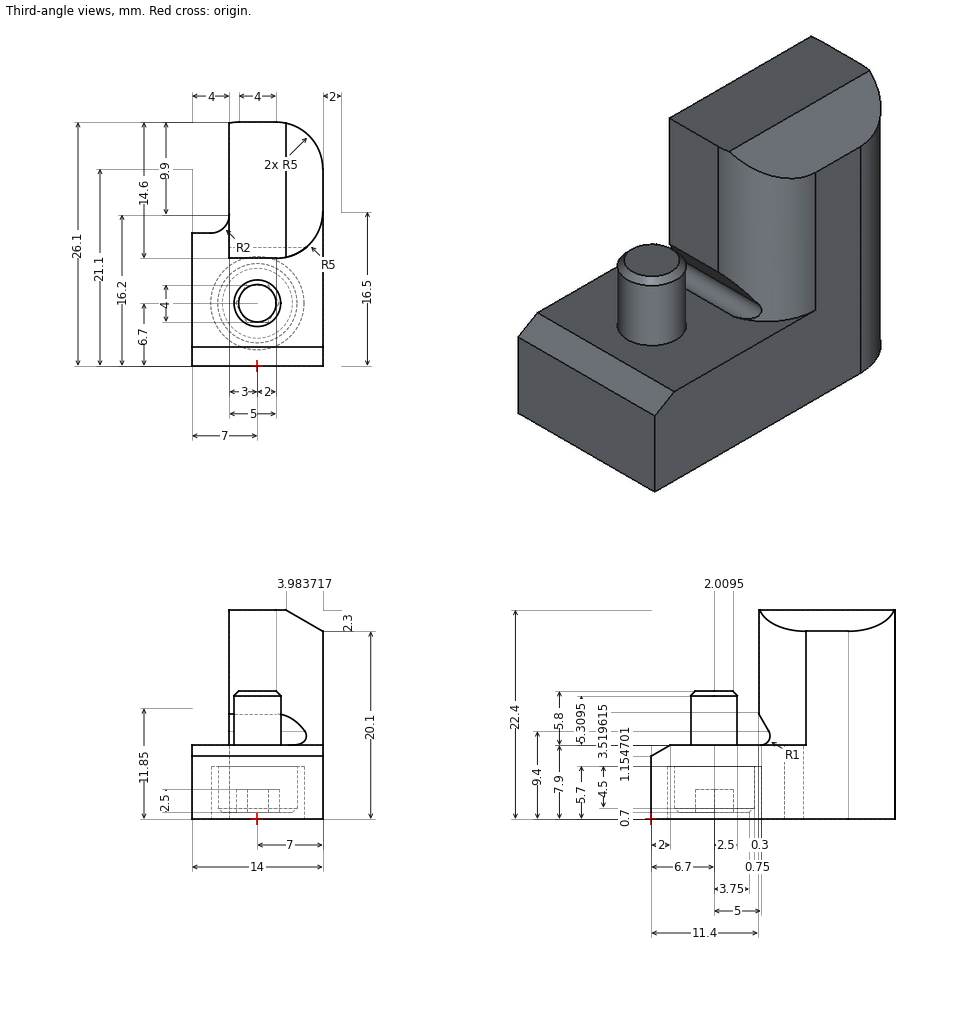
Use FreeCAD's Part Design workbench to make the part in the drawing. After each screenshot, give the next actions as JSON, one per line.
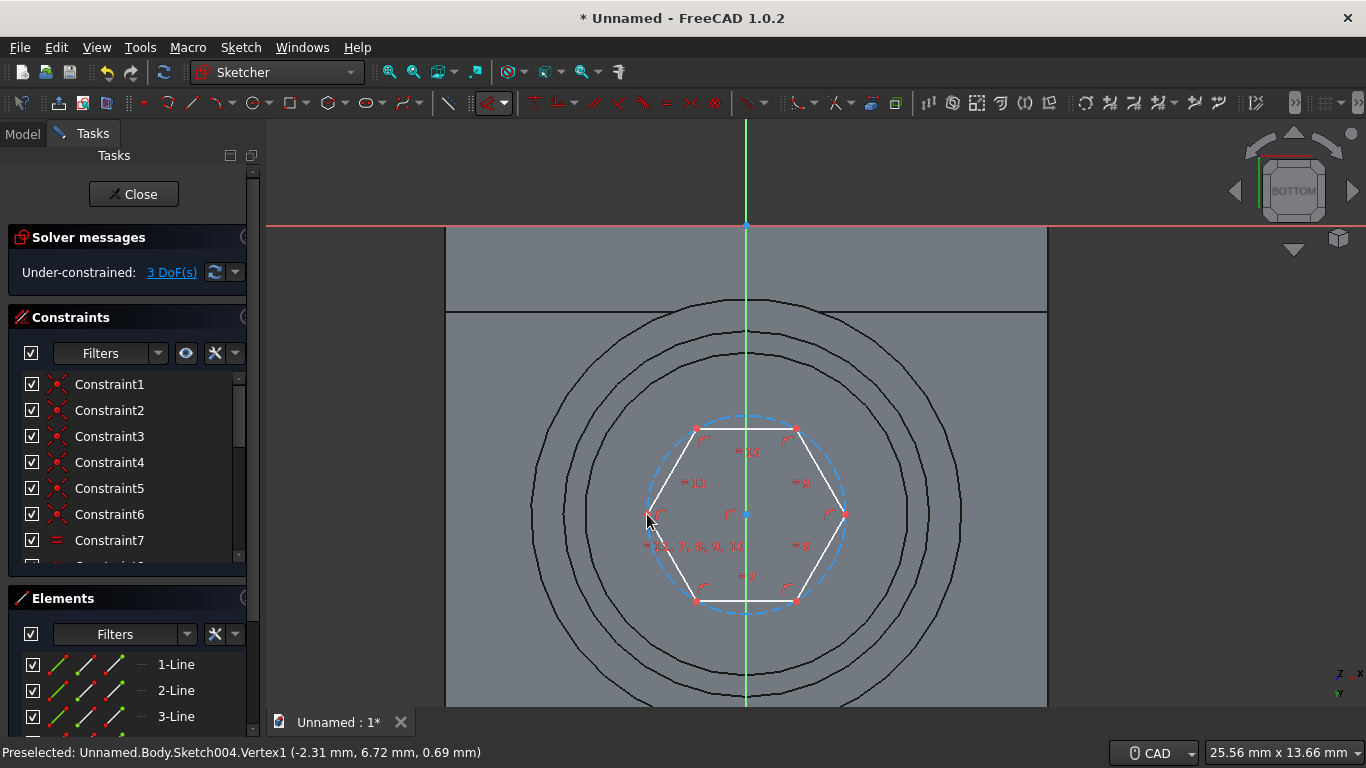
{"action": "scroll", "coordinate": [726, 601], "scroll_direction": "up", "scroll_amount": 2}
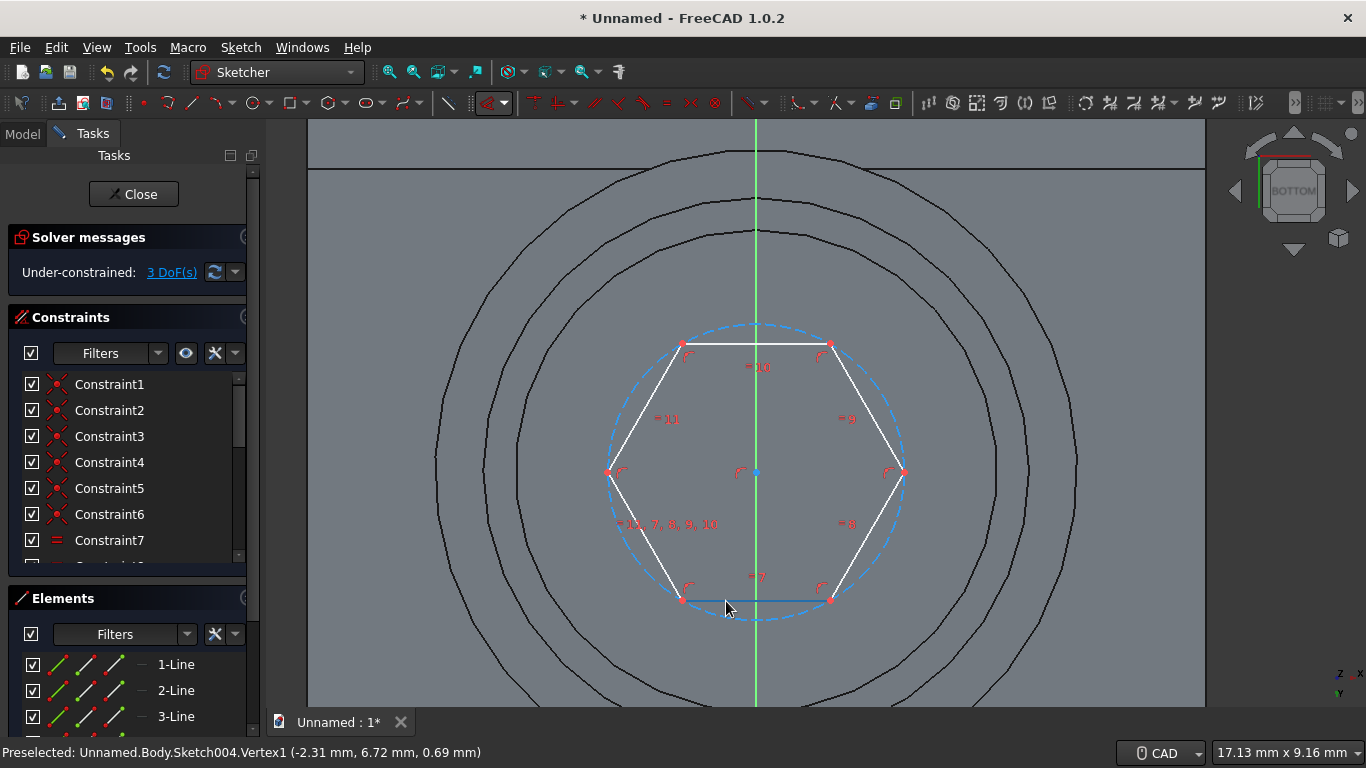
{"action": "left_click", "coordinate": [727, 601]}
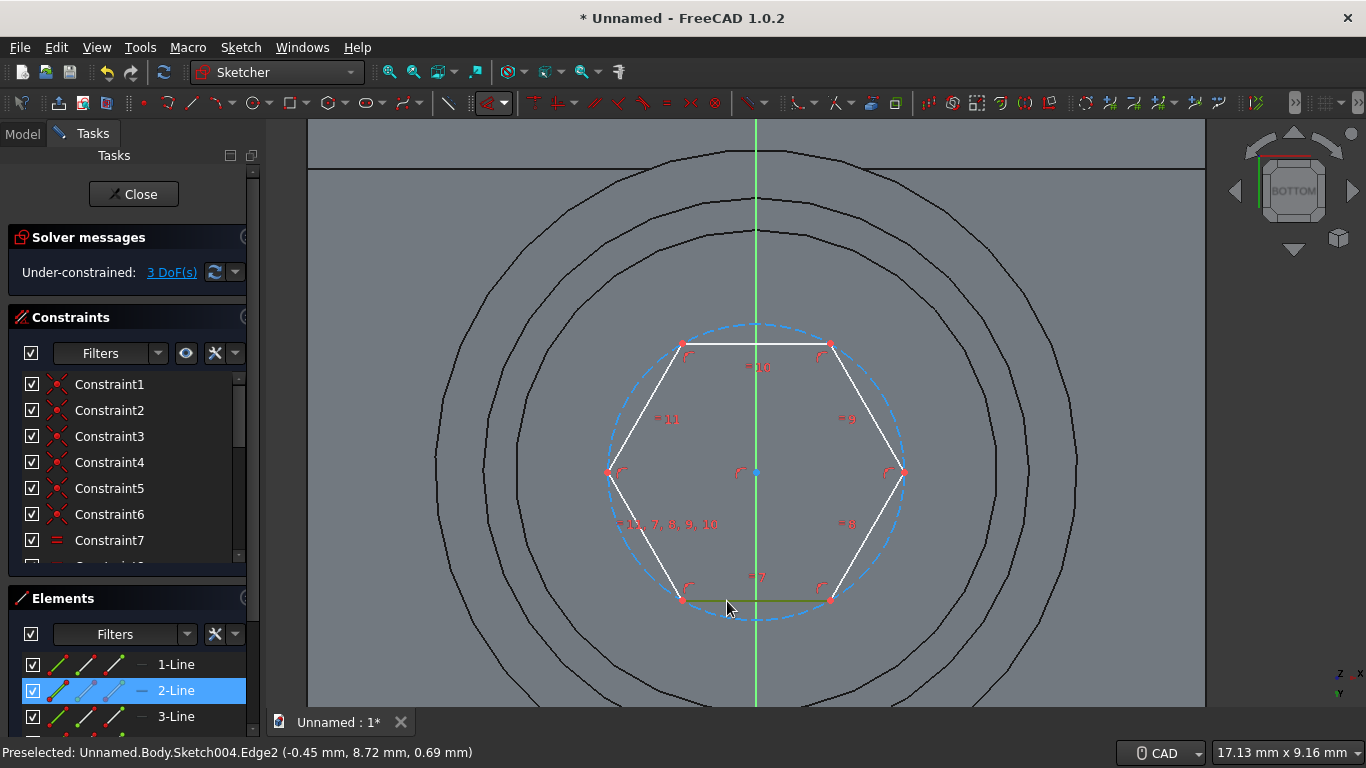
{"action": "key", "text": "h"}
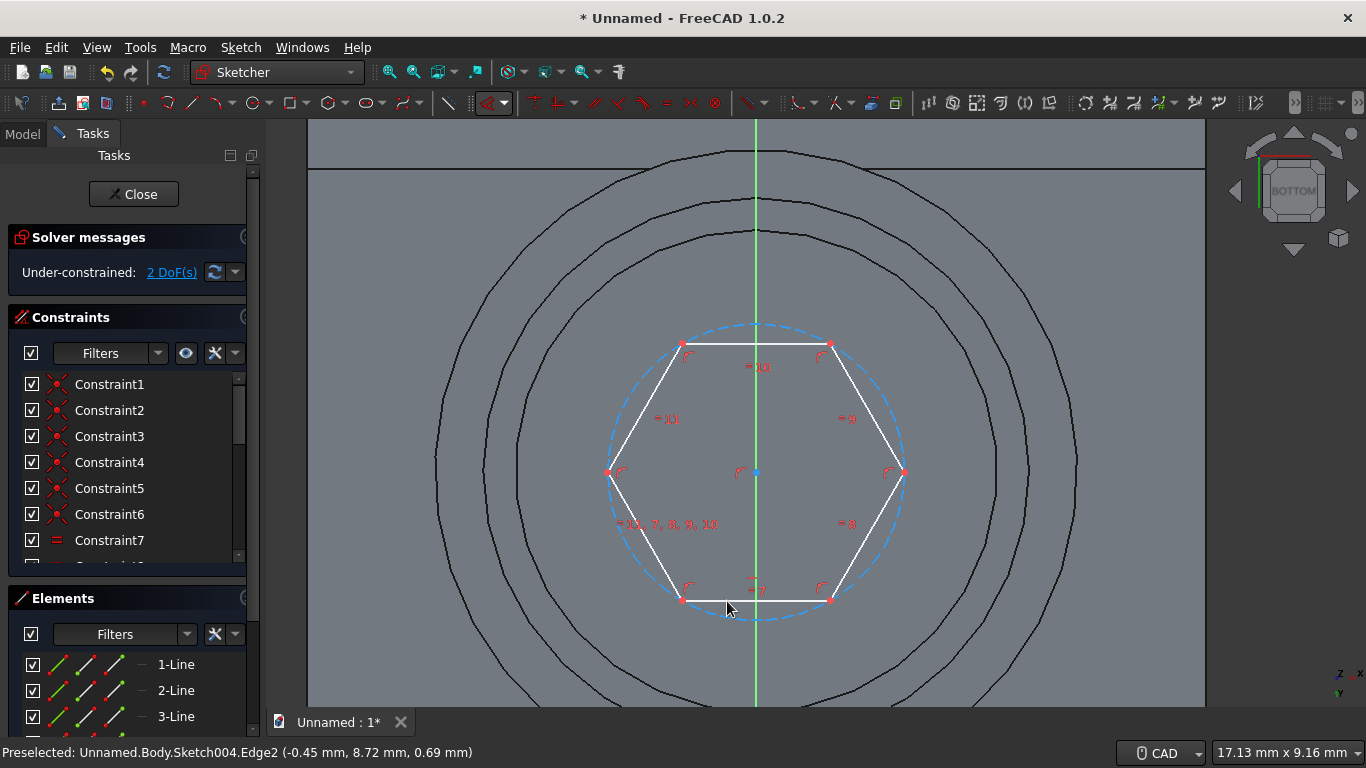
{"action": "left_click", "coordinate": [682, 601]}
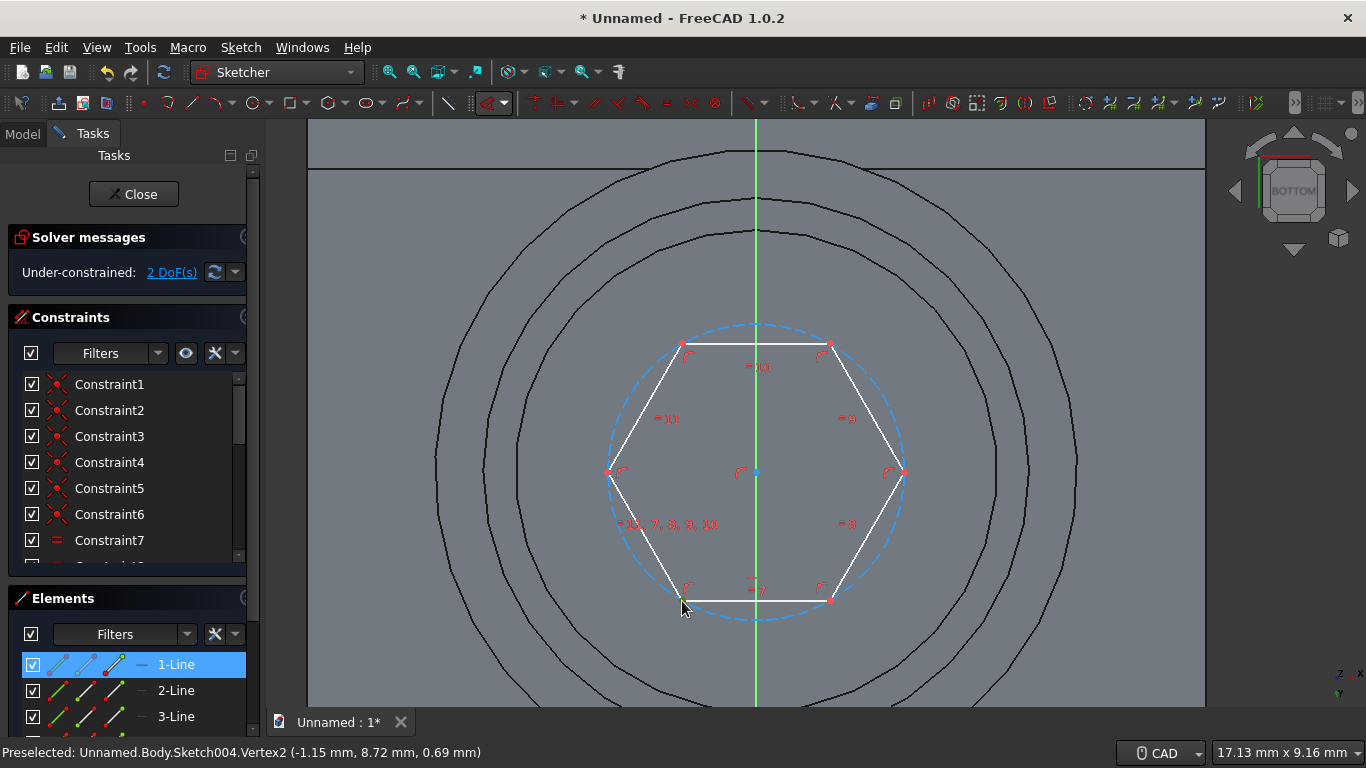
{"action": "left_click", "coordinate": [830, 344]}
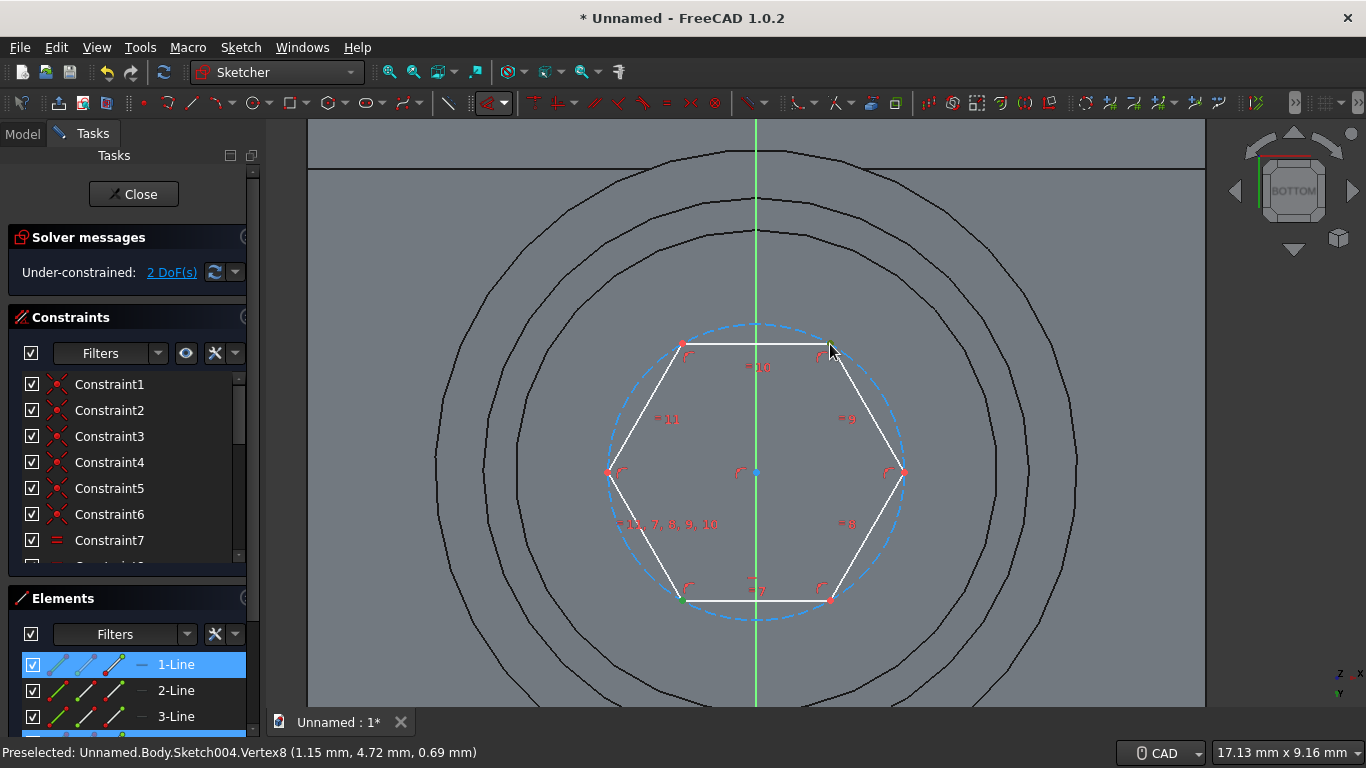
{"action": "left_click", "coordinate": [506, 104]}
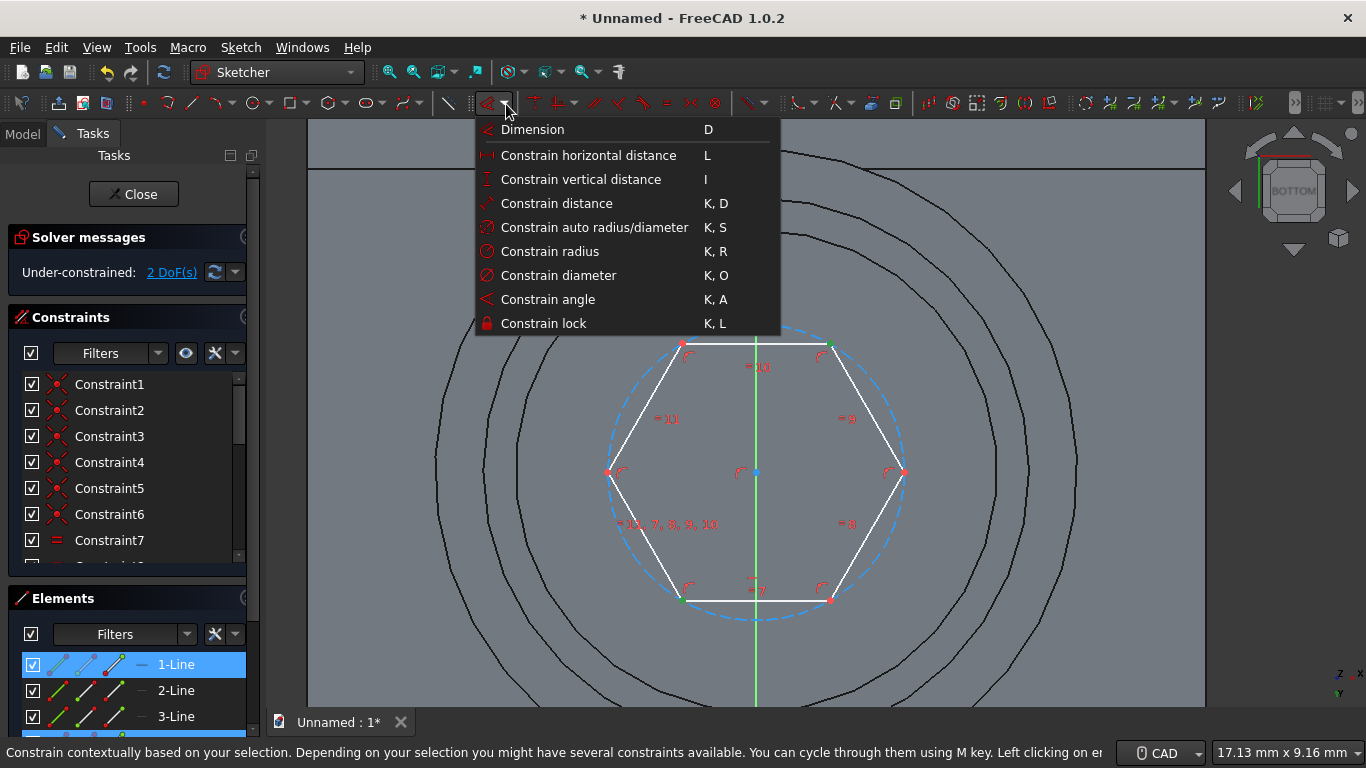
{"action": "left_click", "coordinate": [628, 179]}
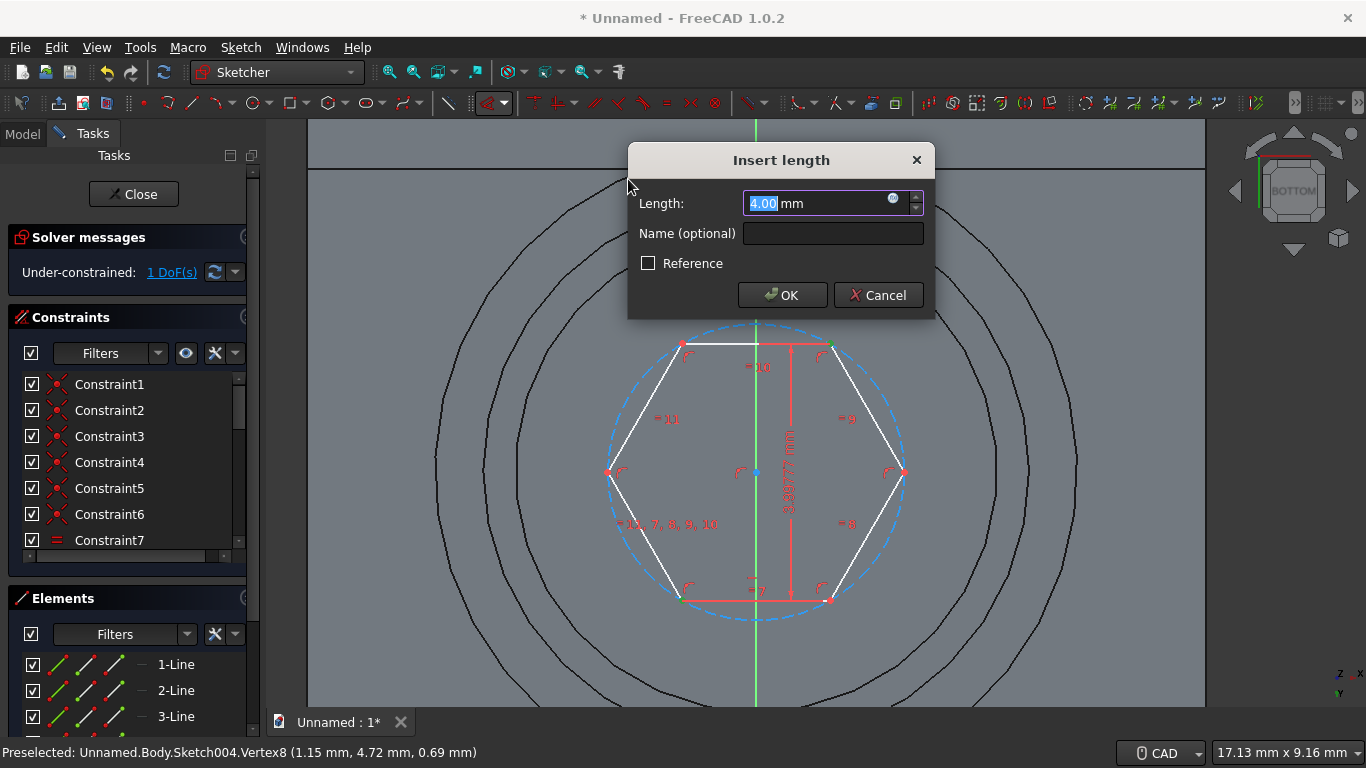
{"action": "type", "text": "4"}
{"action": "key", "text": "Return"}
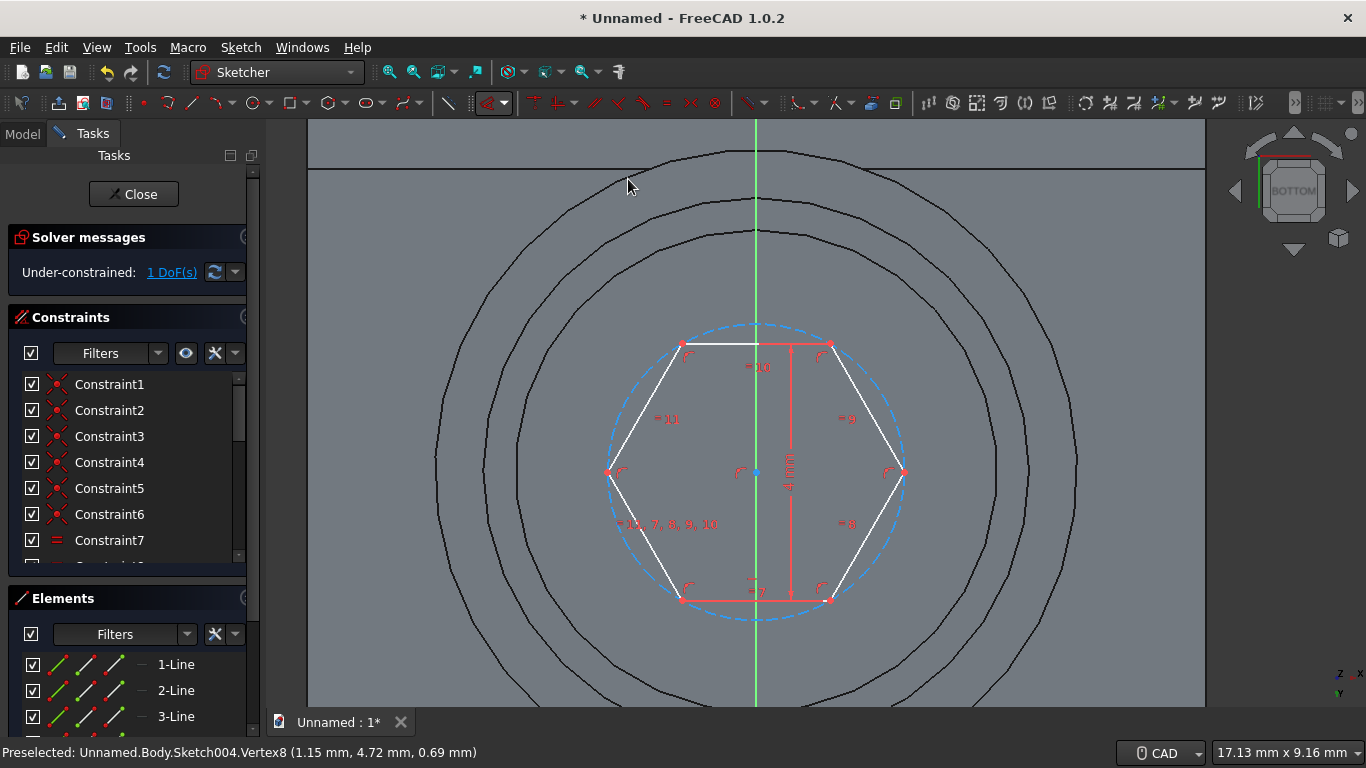
{"action": "left_click", "coordinate": [756, 472]}